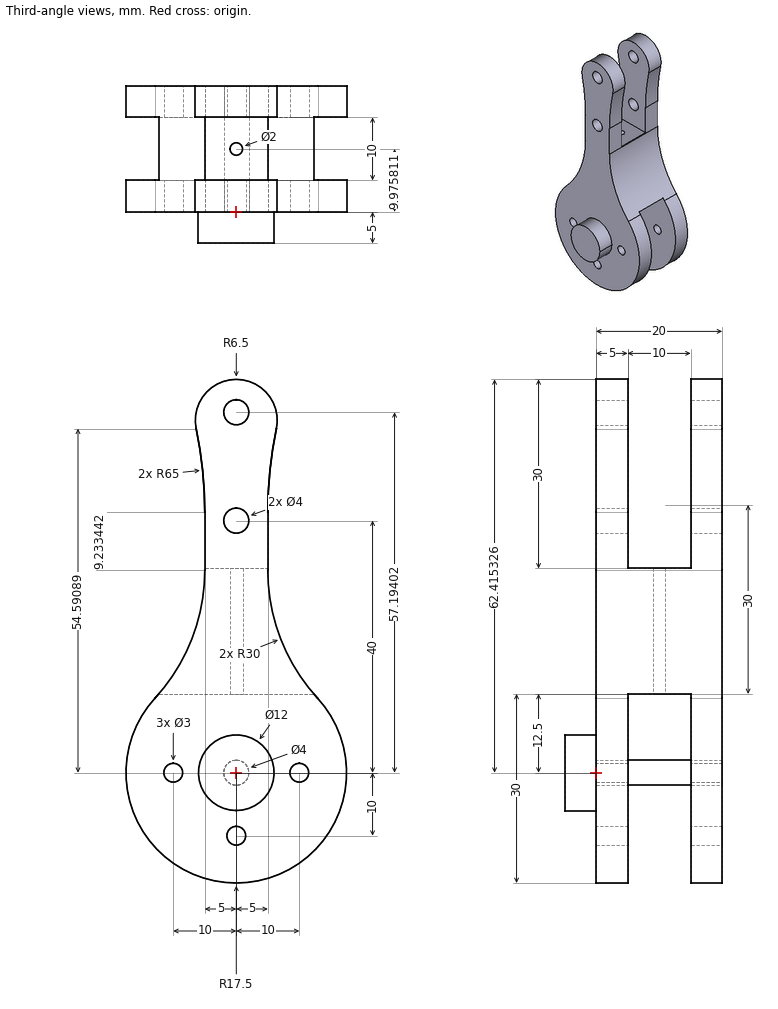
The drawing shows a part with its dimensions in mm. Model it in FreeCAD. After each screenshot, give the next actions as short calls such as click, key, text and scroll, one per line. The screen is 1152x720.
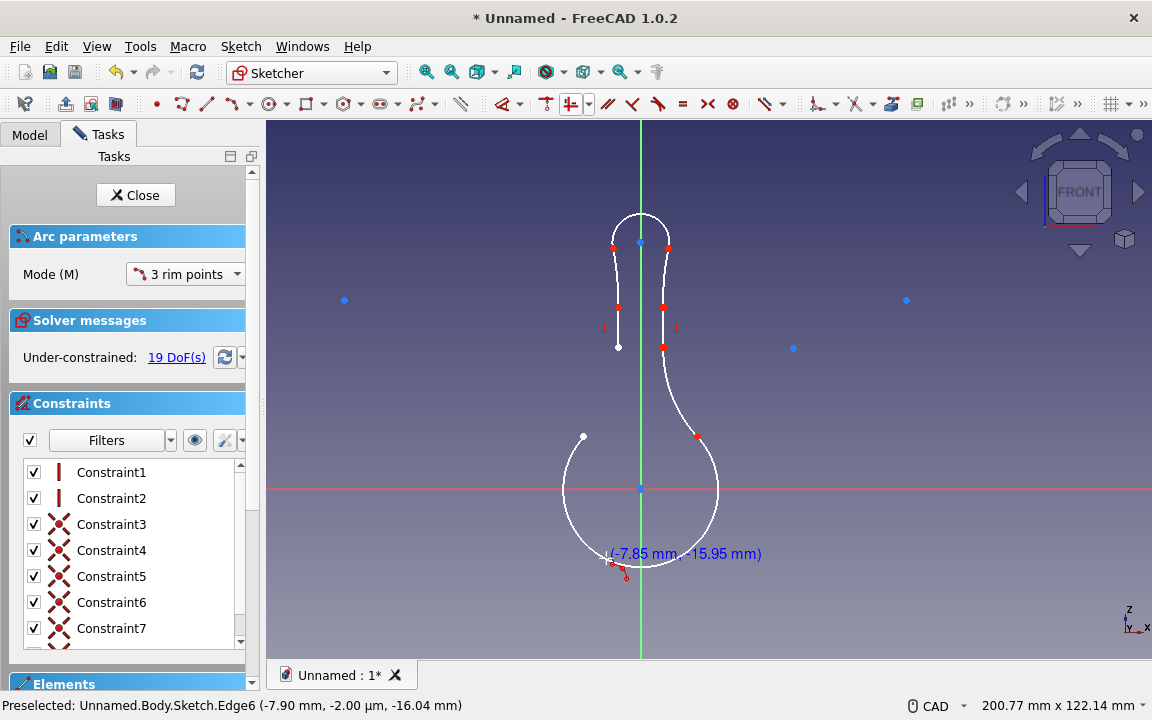
click(584, 437)
click(618, 348)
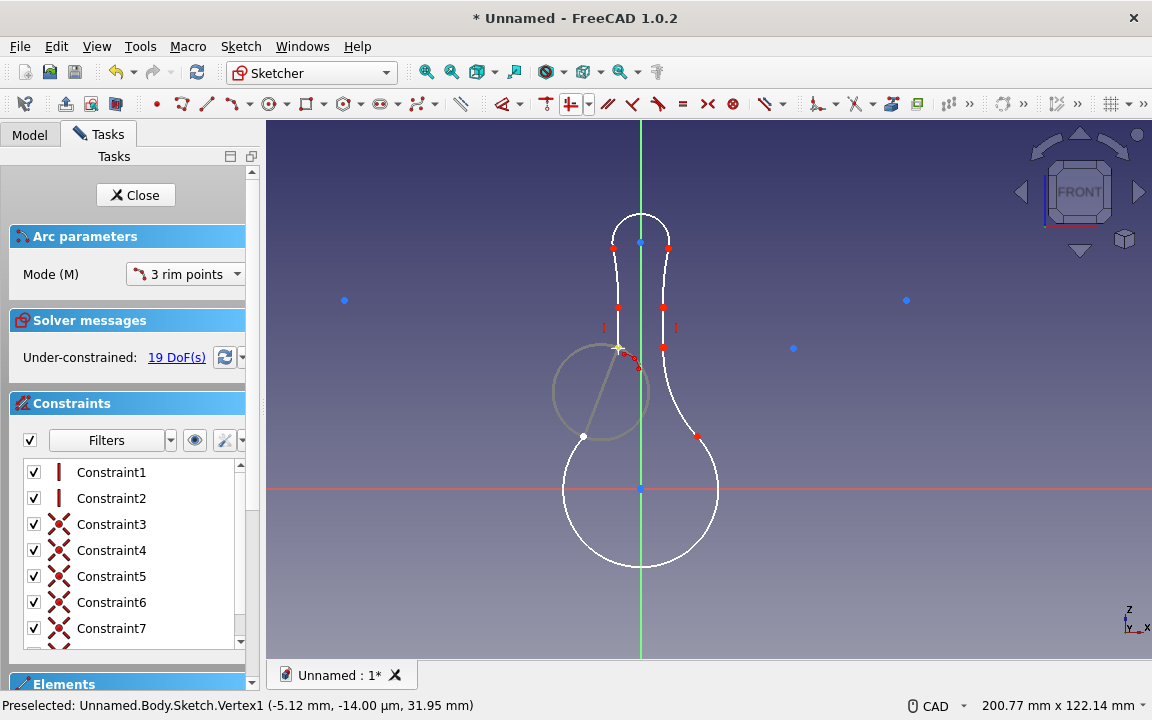
scroll(610, 395, up, 3)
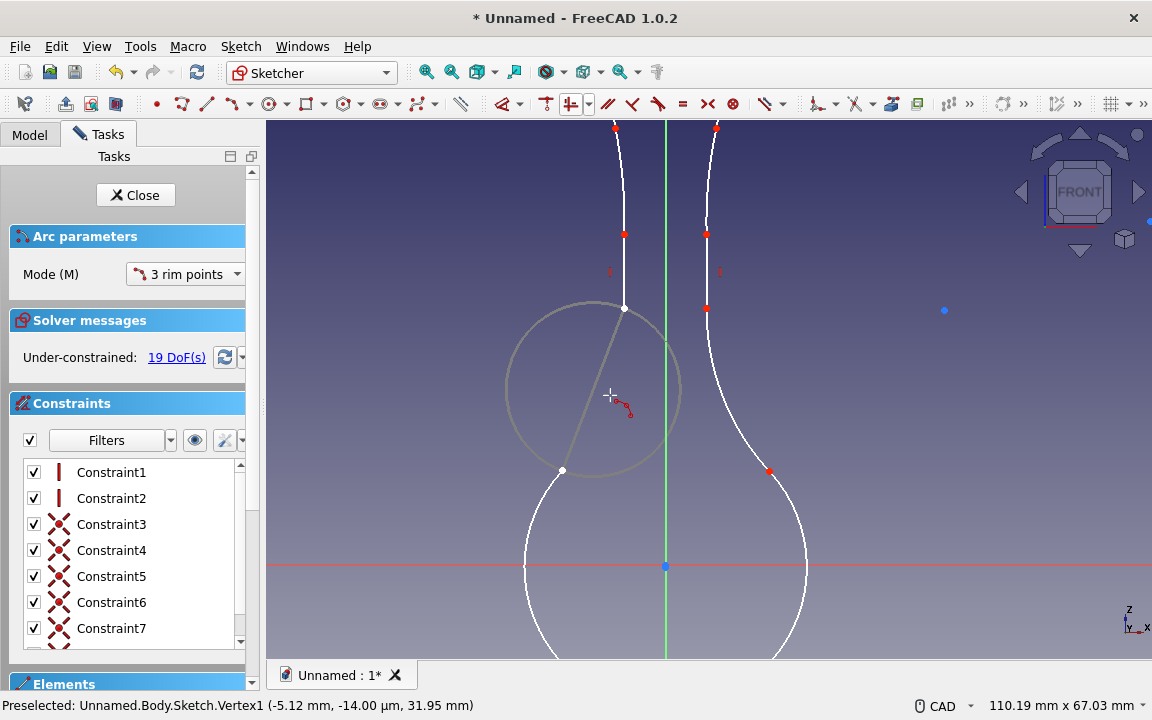
click(609, 394)
key(Escape)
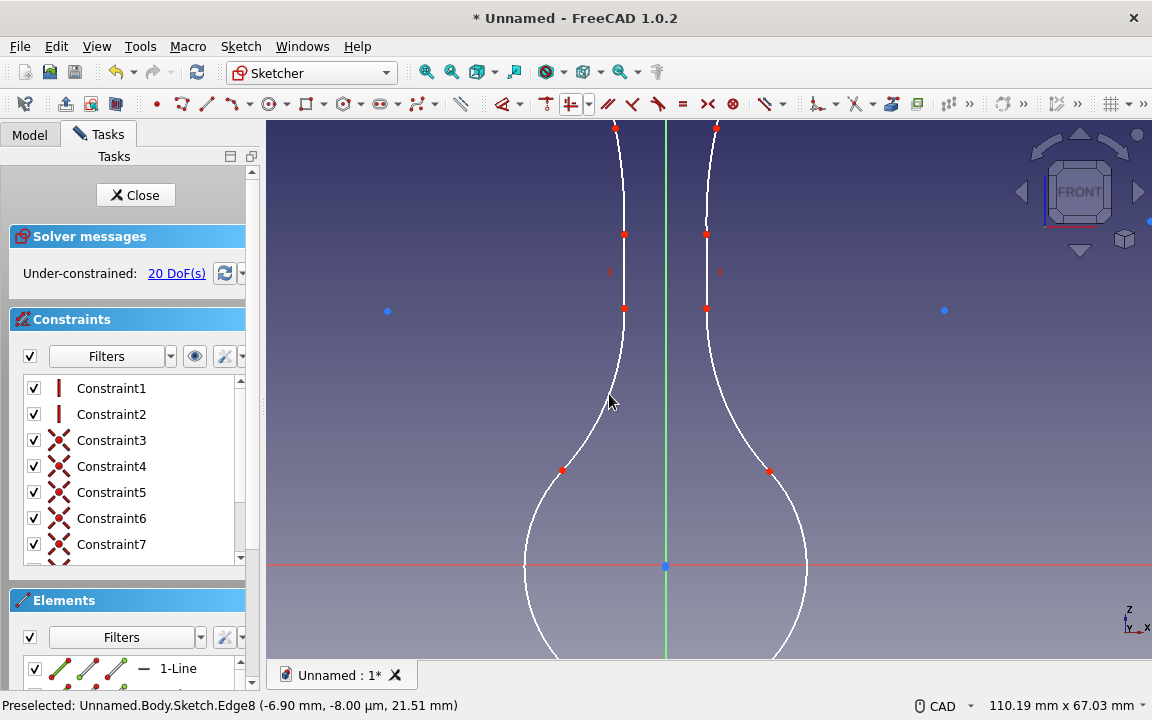
click(624, 286)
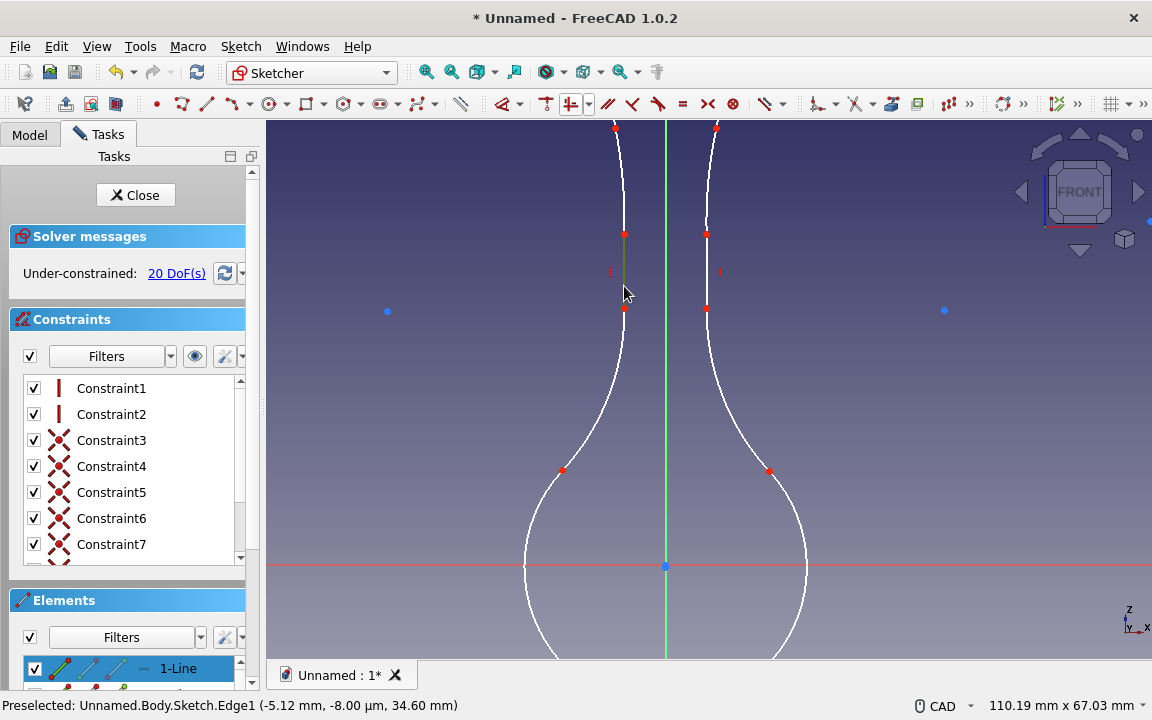
click(594, 428)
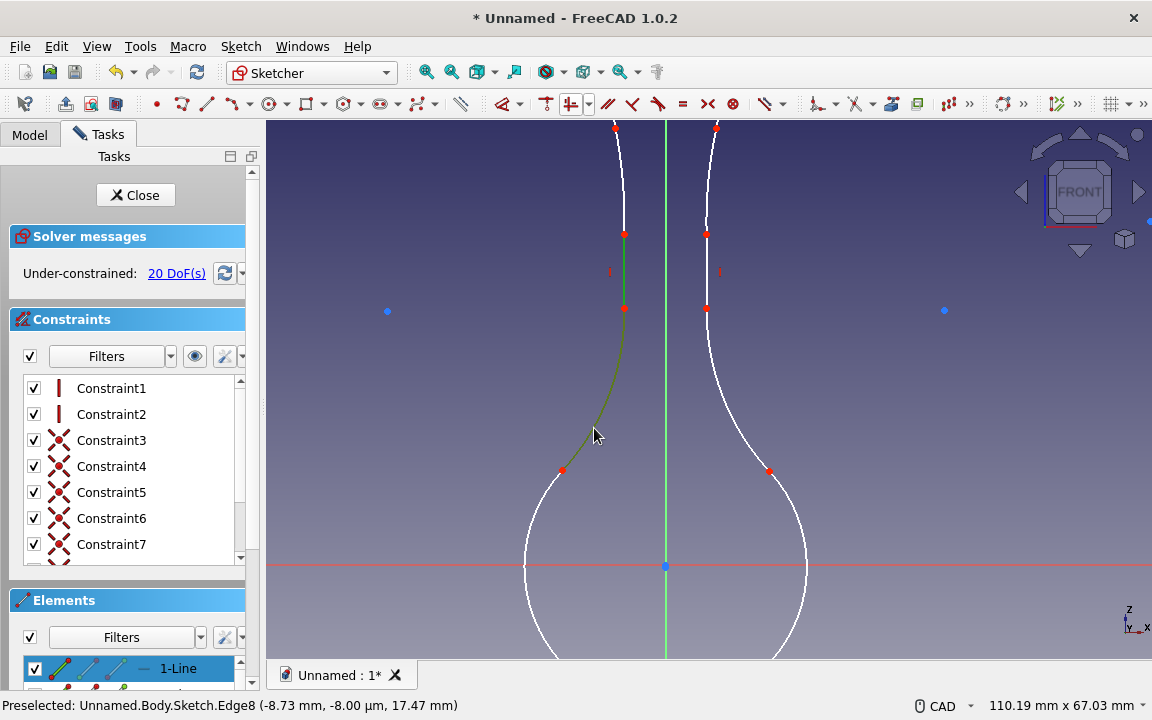
click(658, 104)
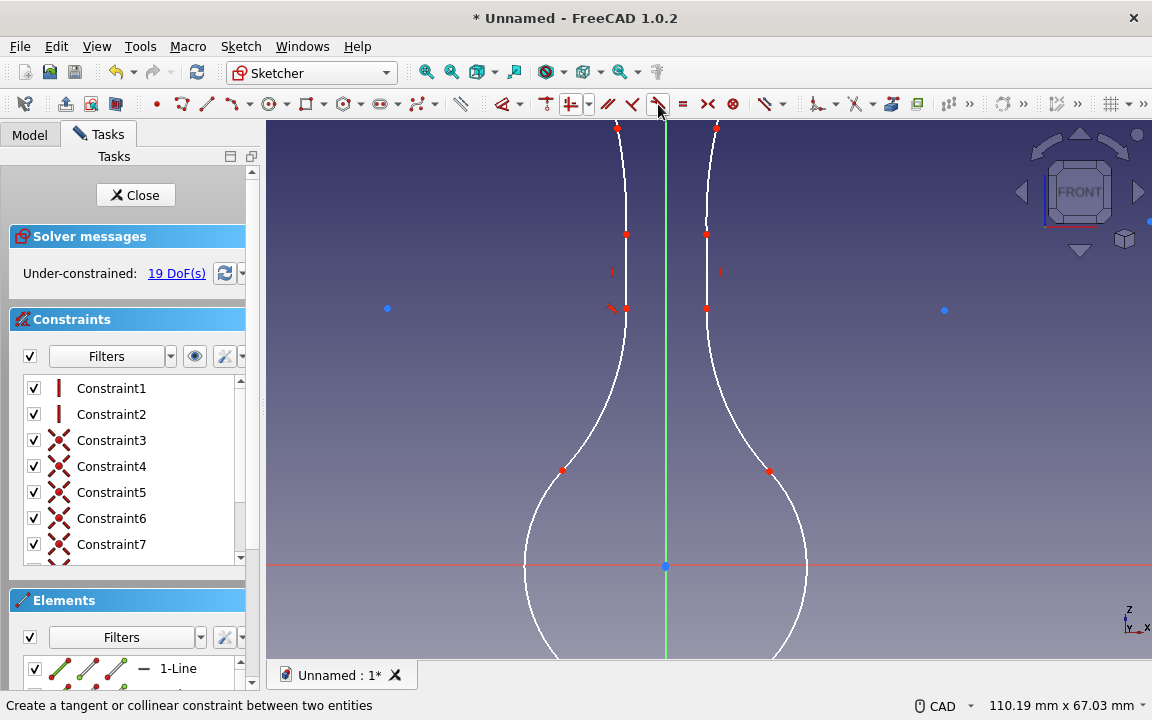
click(707, 257)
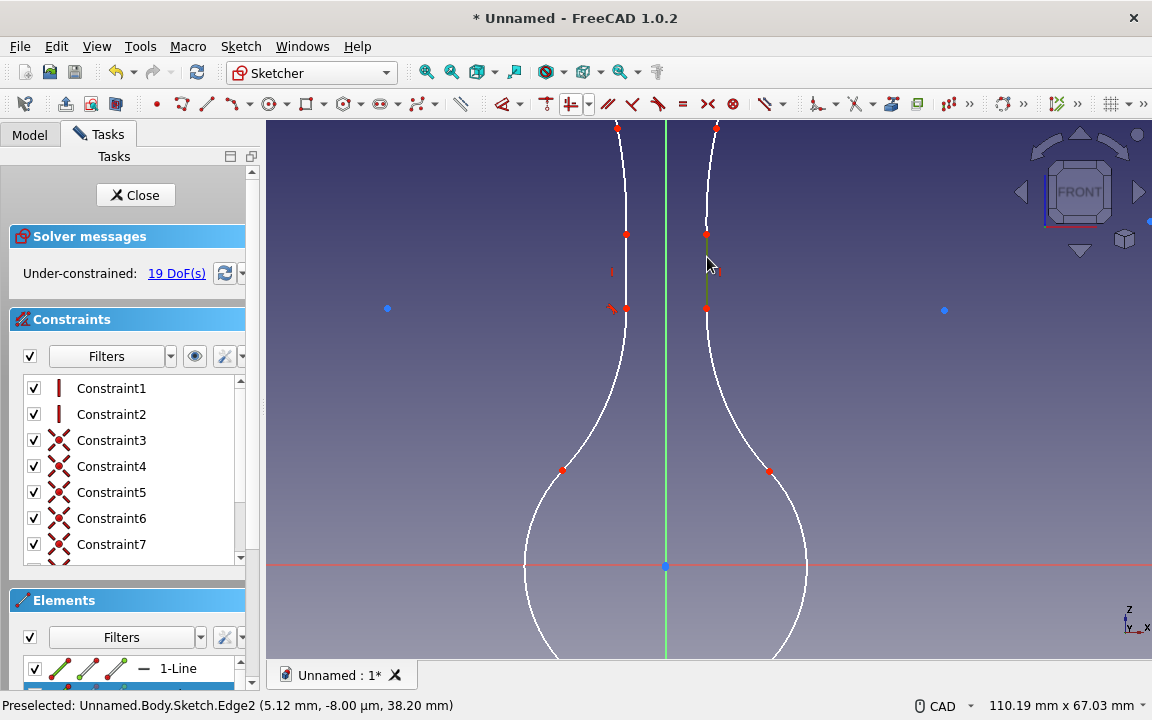
click(712, 361)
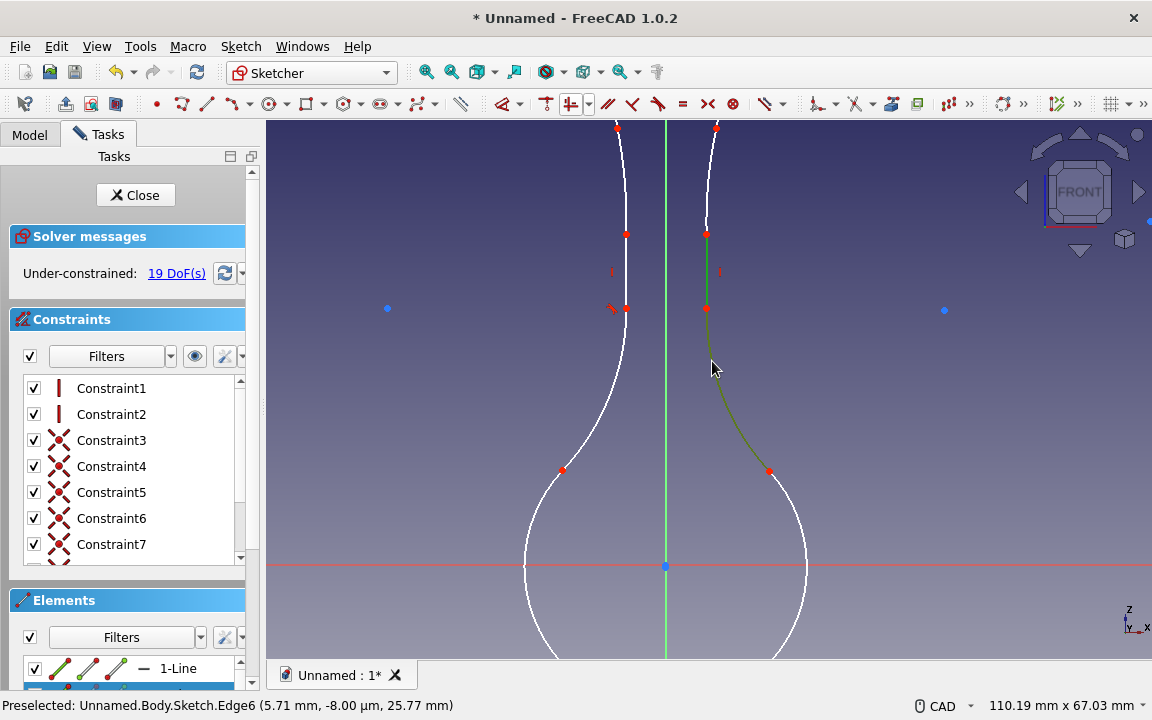
click(658, 104)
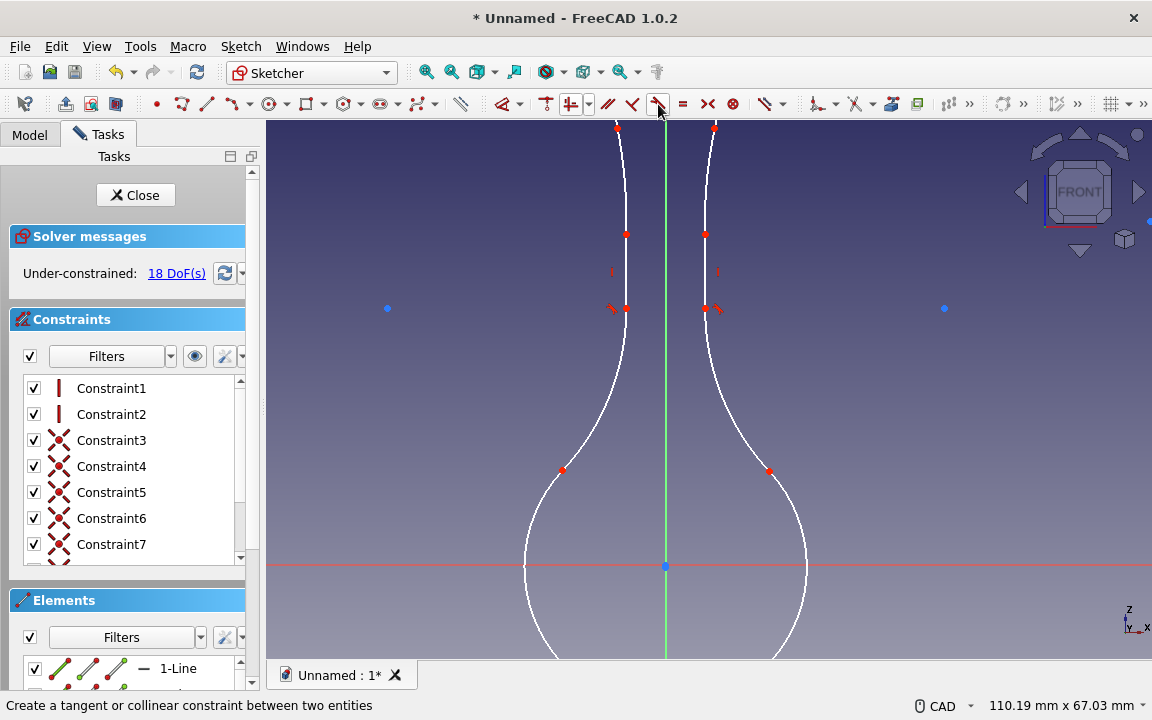
click(626, 203)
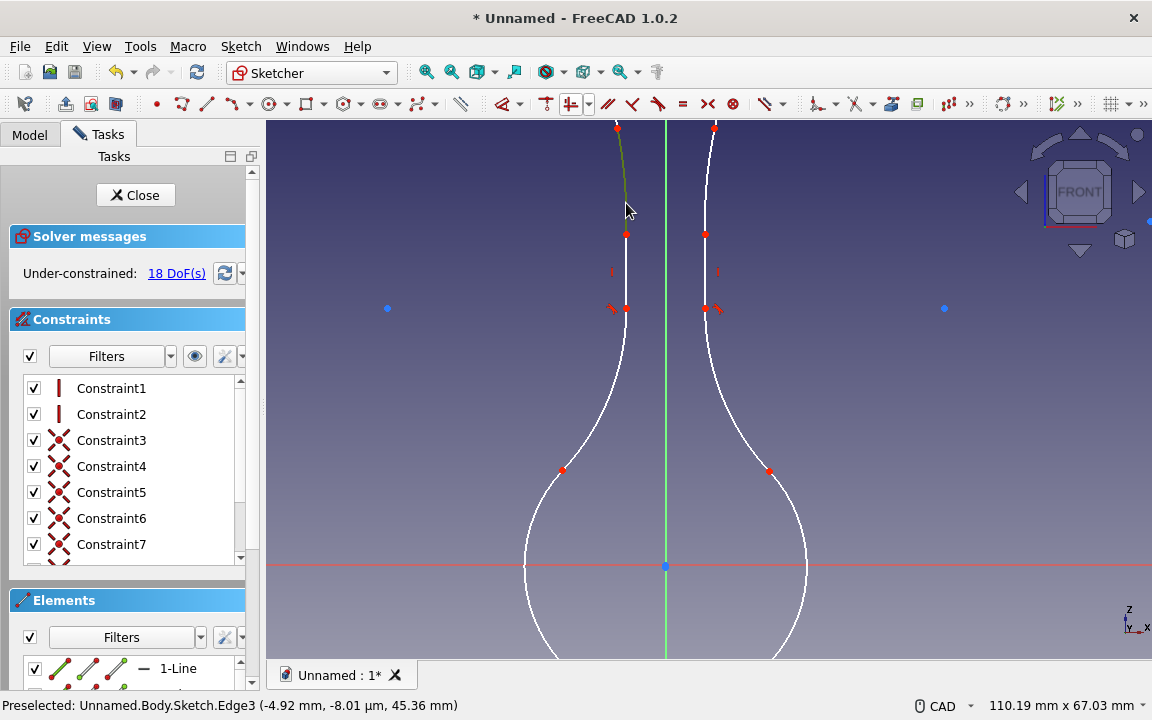
scroll(610, 395, down, 3)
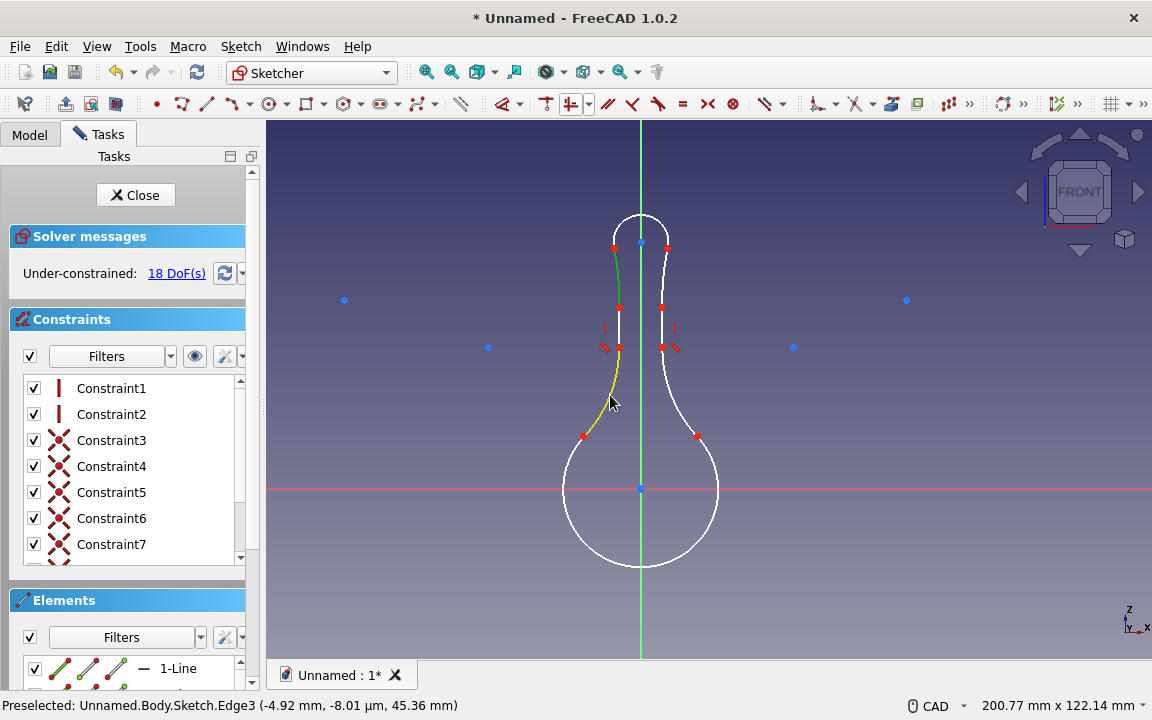
click(659, 222)